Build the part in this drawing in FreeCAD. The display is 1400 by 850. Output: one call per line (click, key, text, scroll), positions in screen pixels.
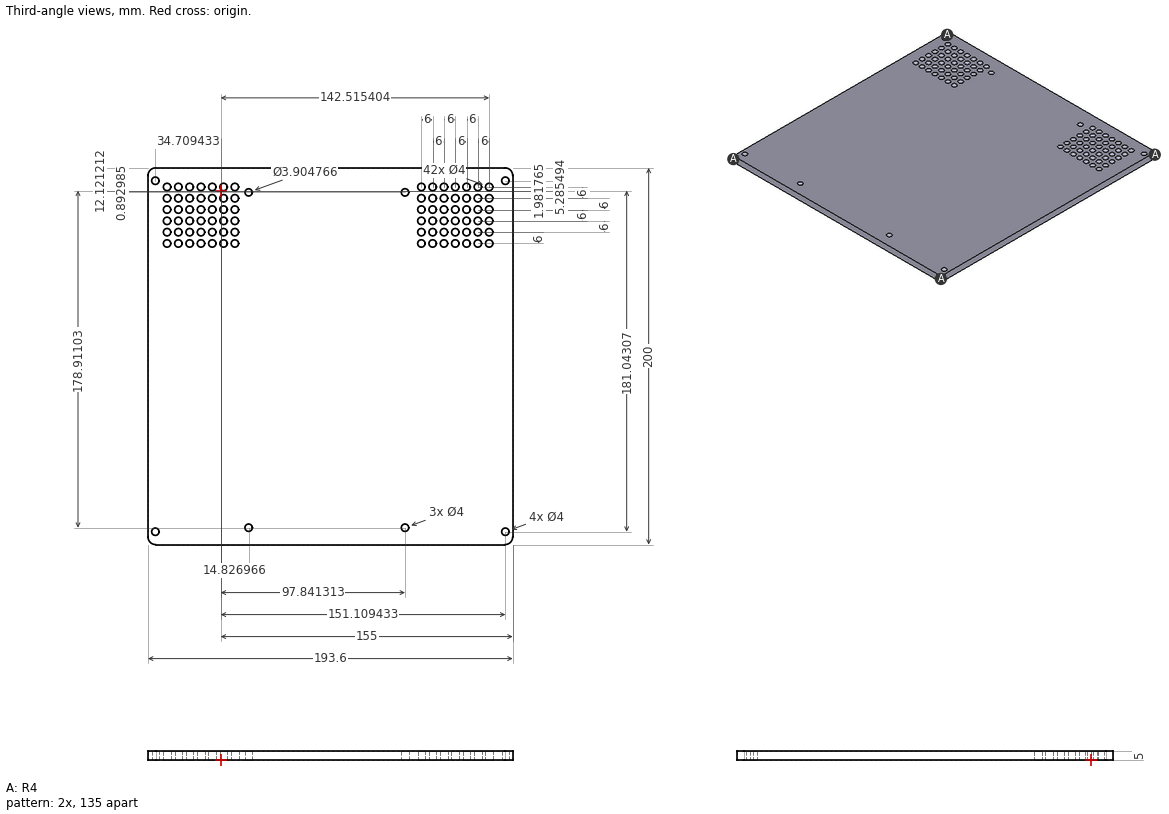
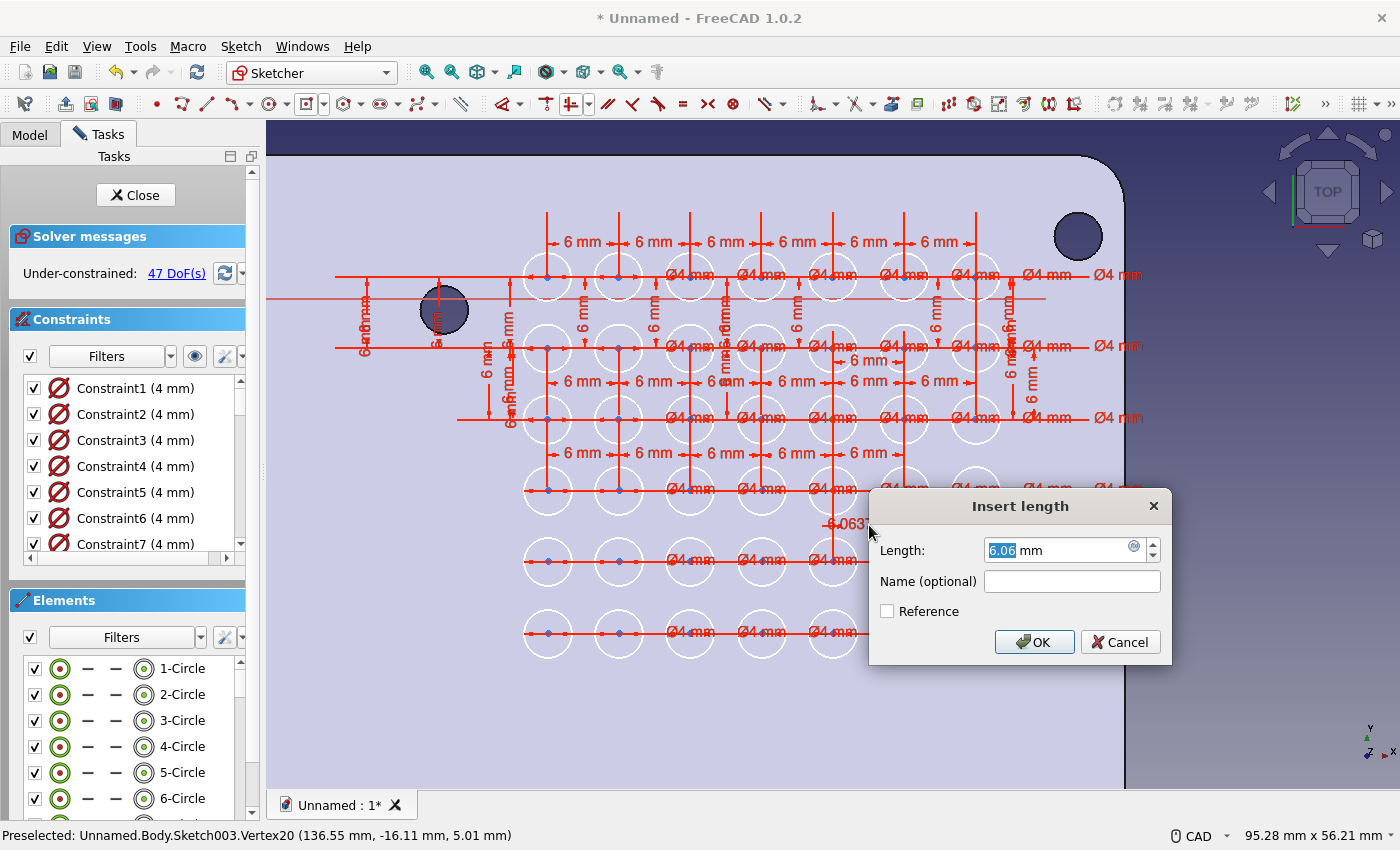
text(6)
key(Return)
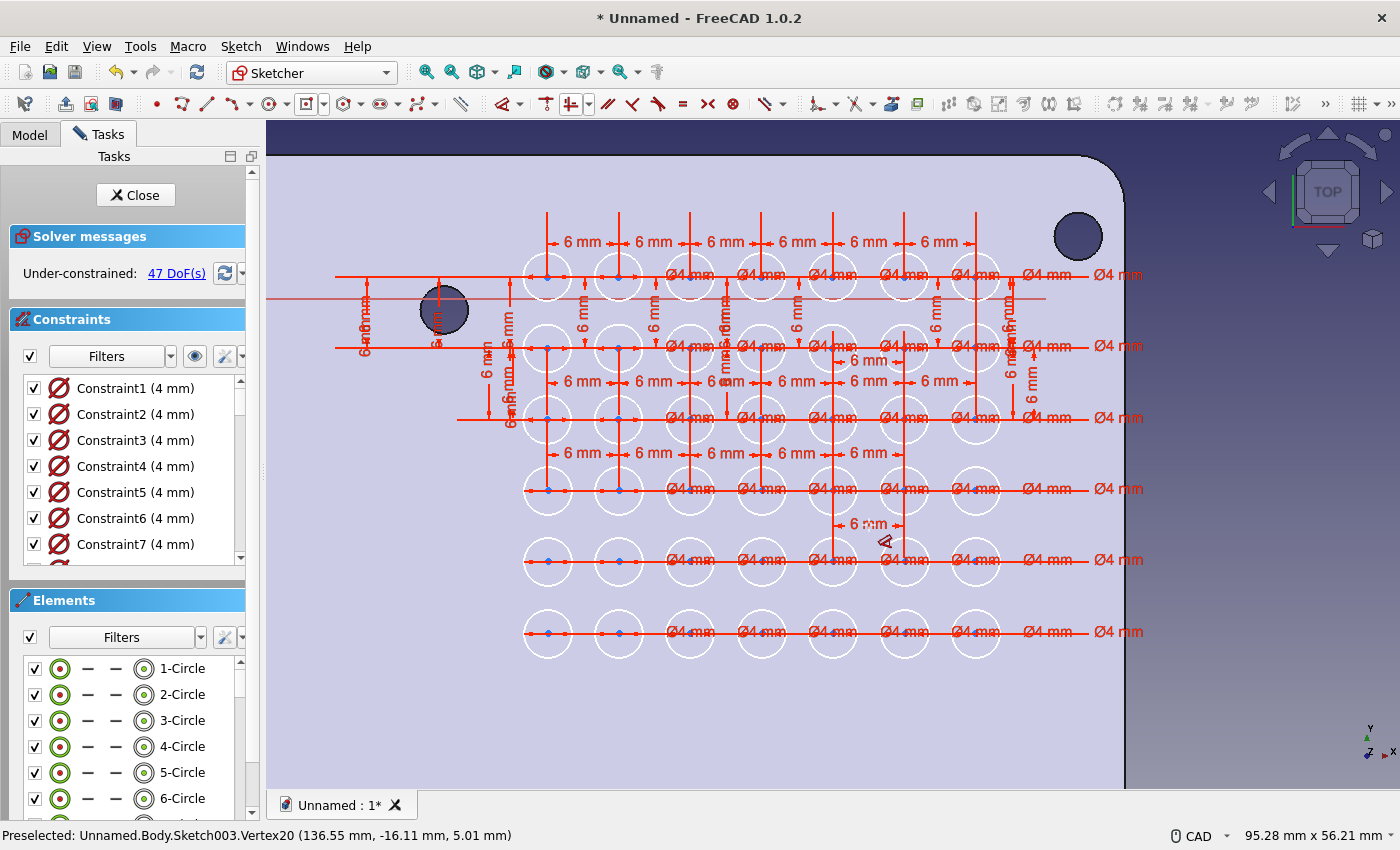
click(904, 420)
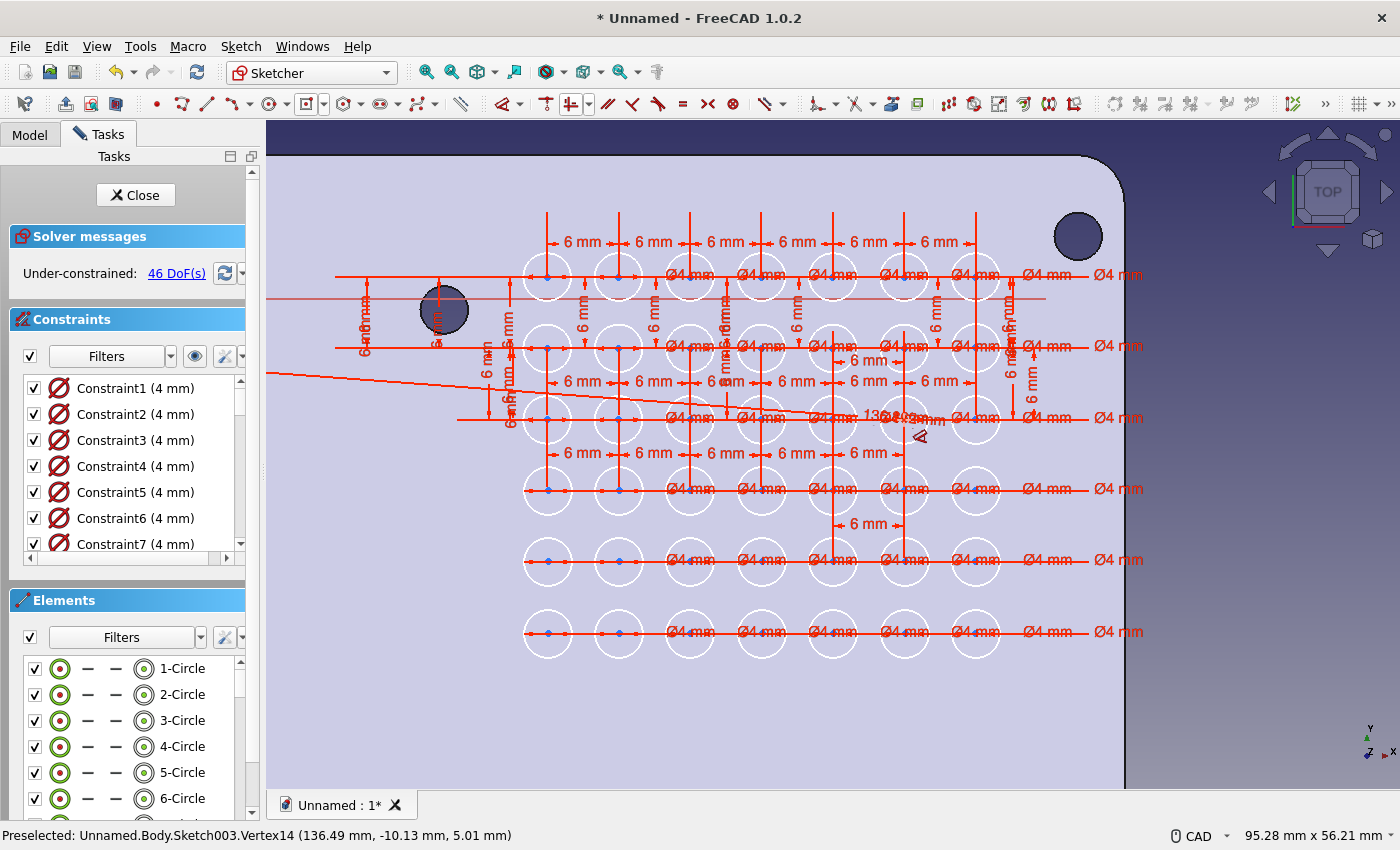
click(904, 491)
click(962, 455)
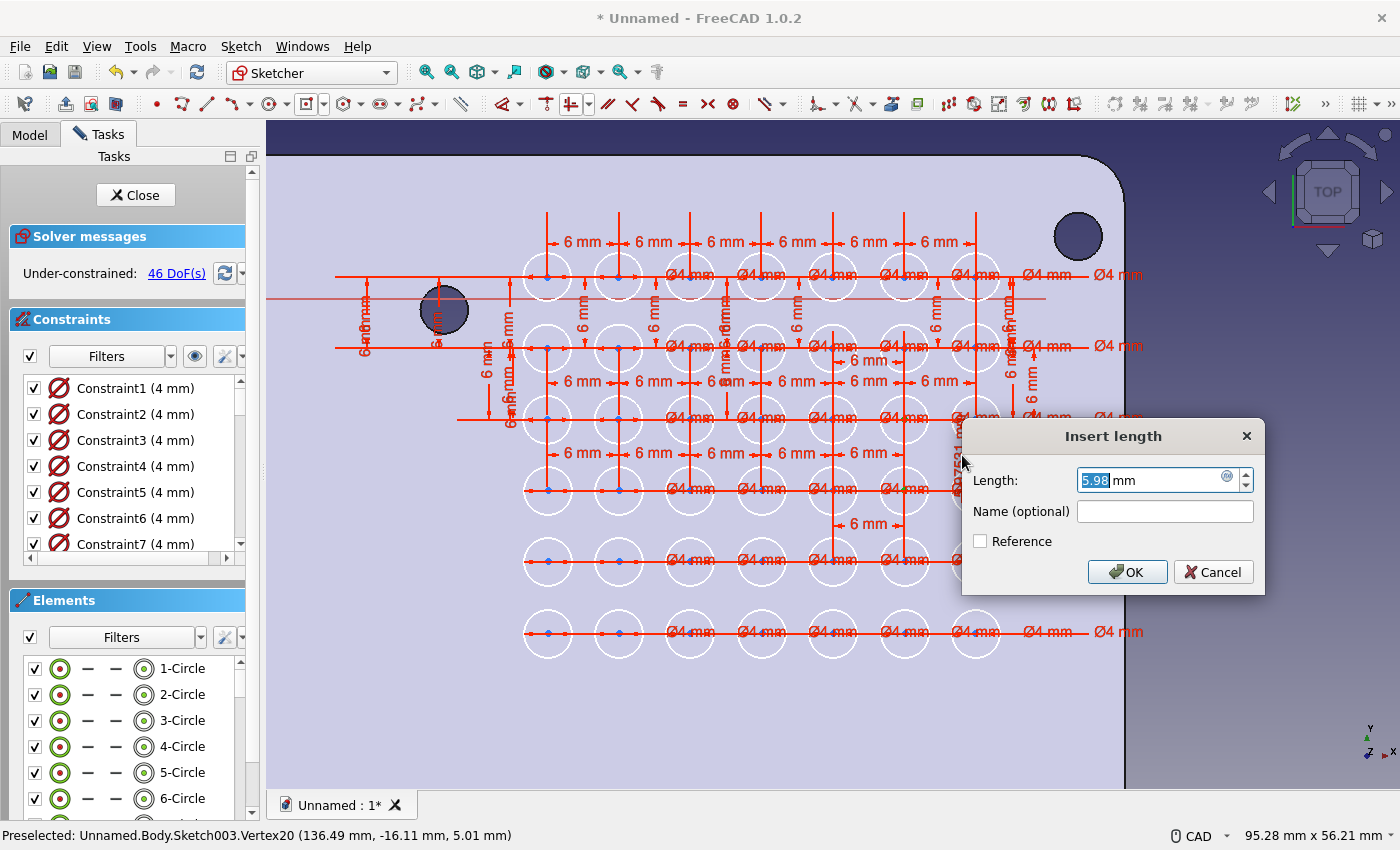
text(6)
key(Return)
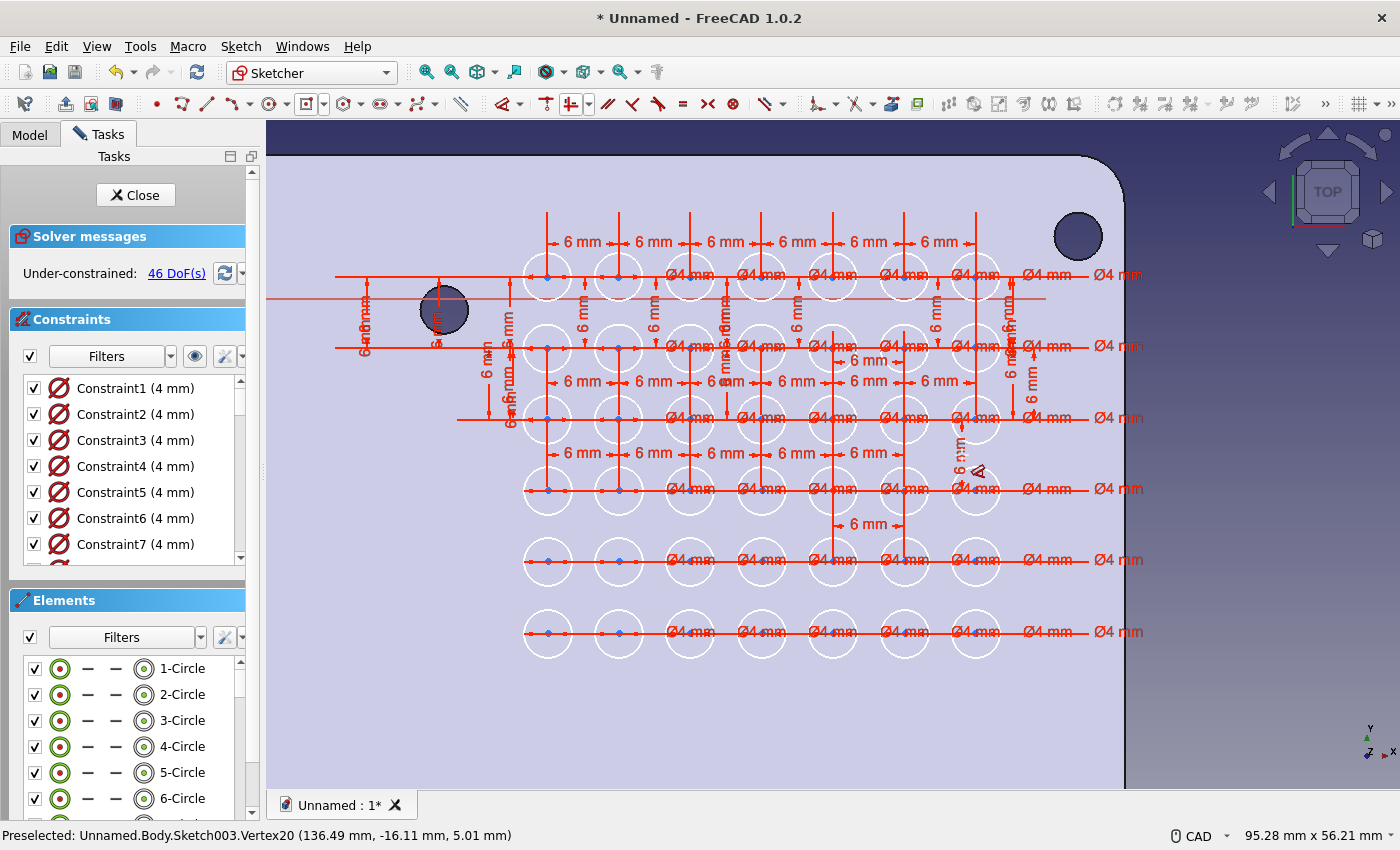
click(904, 491)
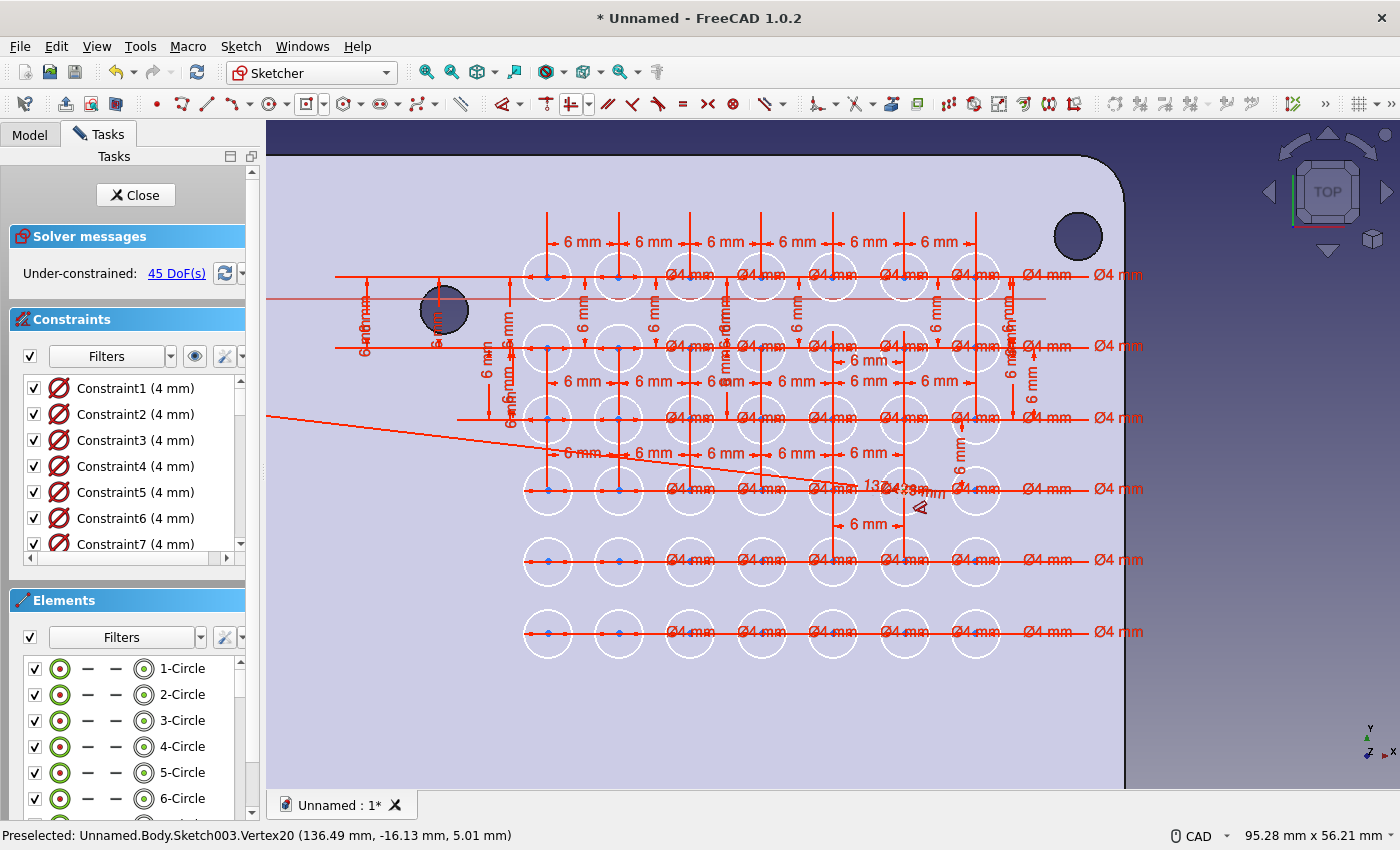
click(833, 491)
click(869, 549)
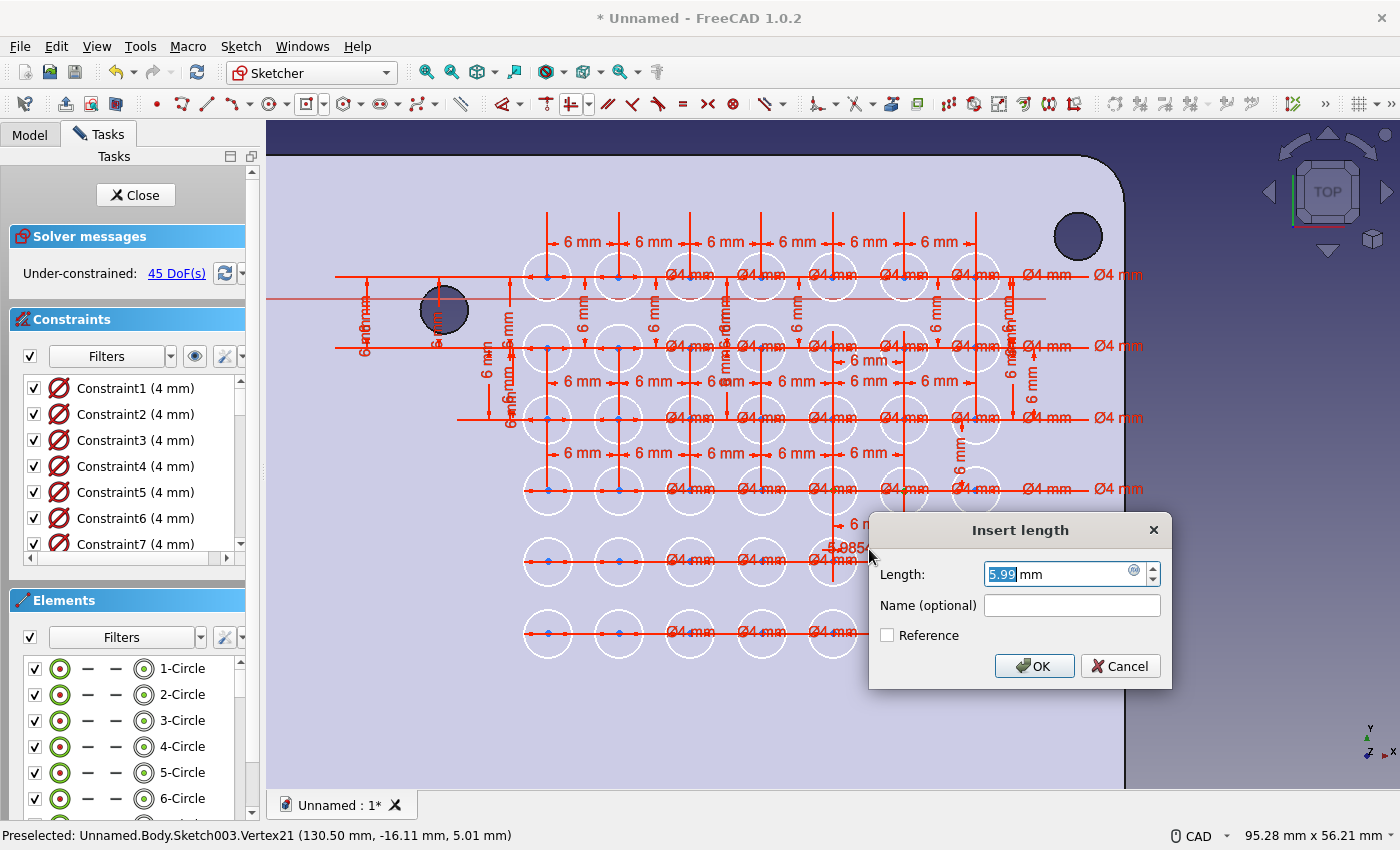
text(6)
key(Return)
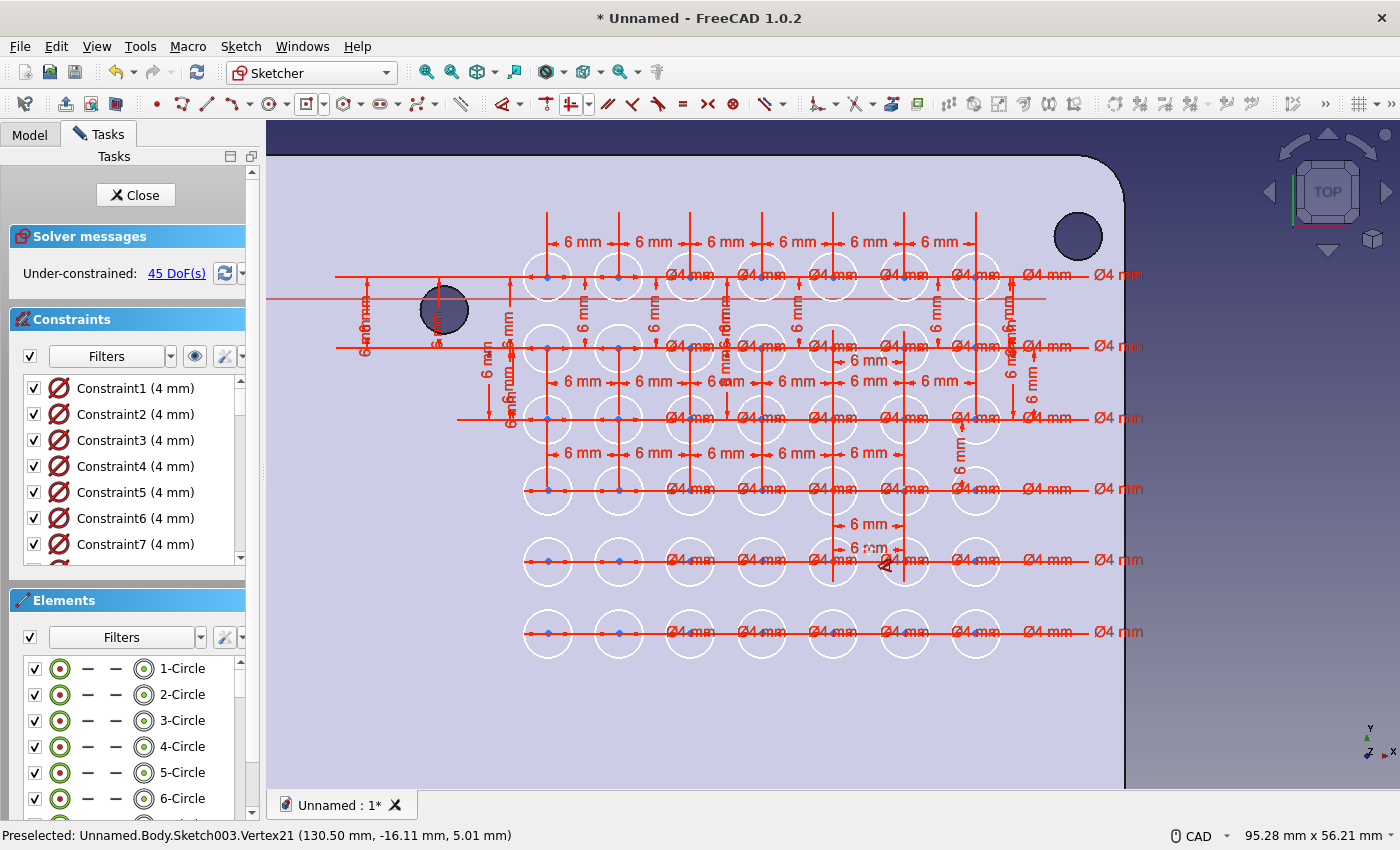
click(833, 420)